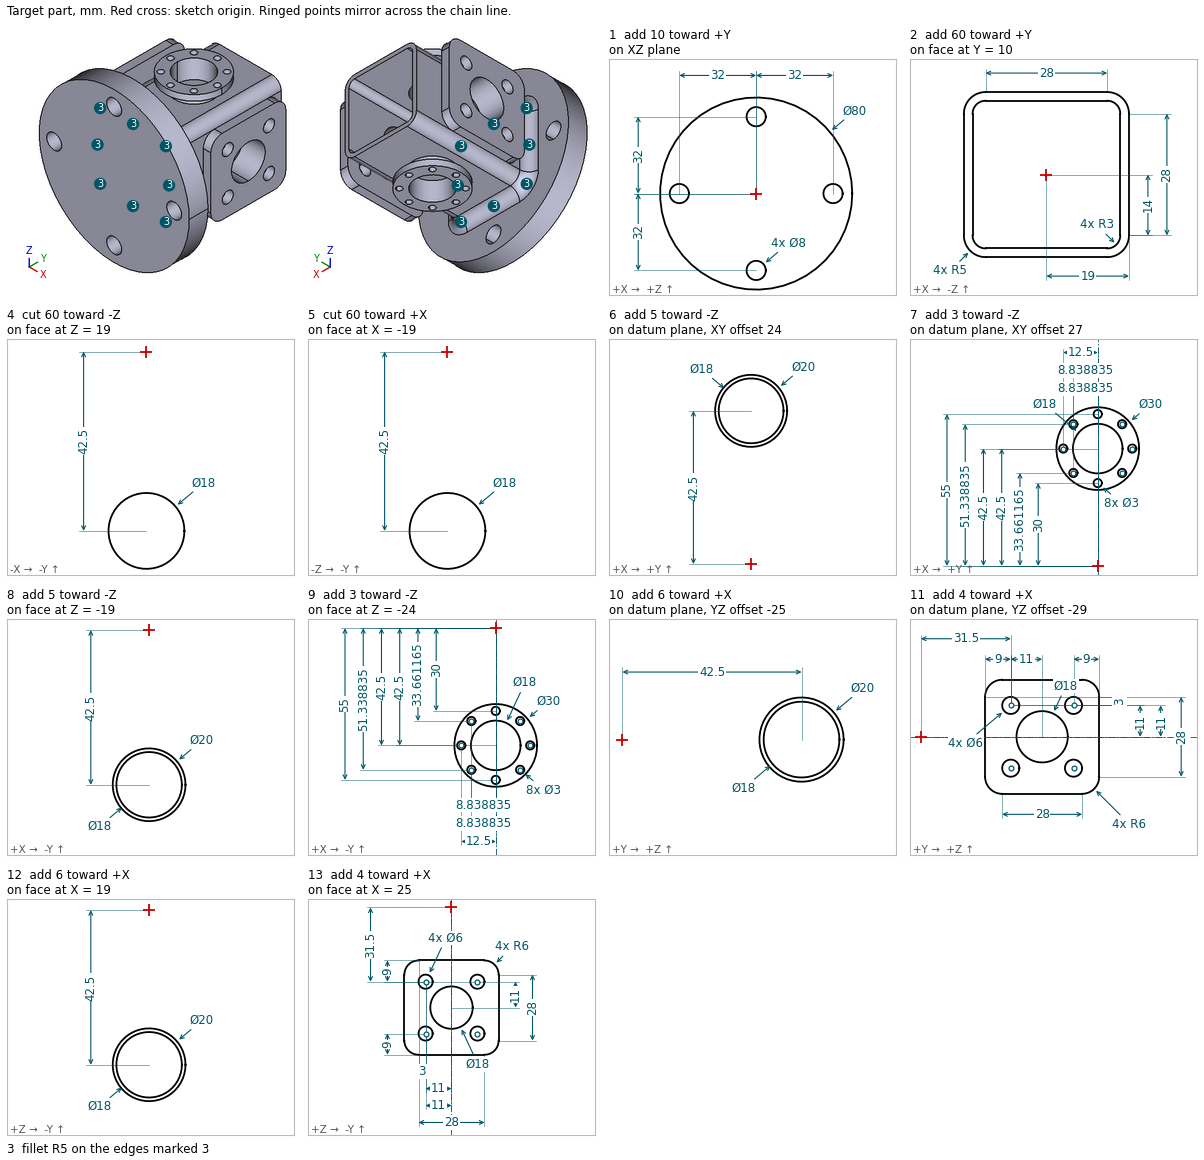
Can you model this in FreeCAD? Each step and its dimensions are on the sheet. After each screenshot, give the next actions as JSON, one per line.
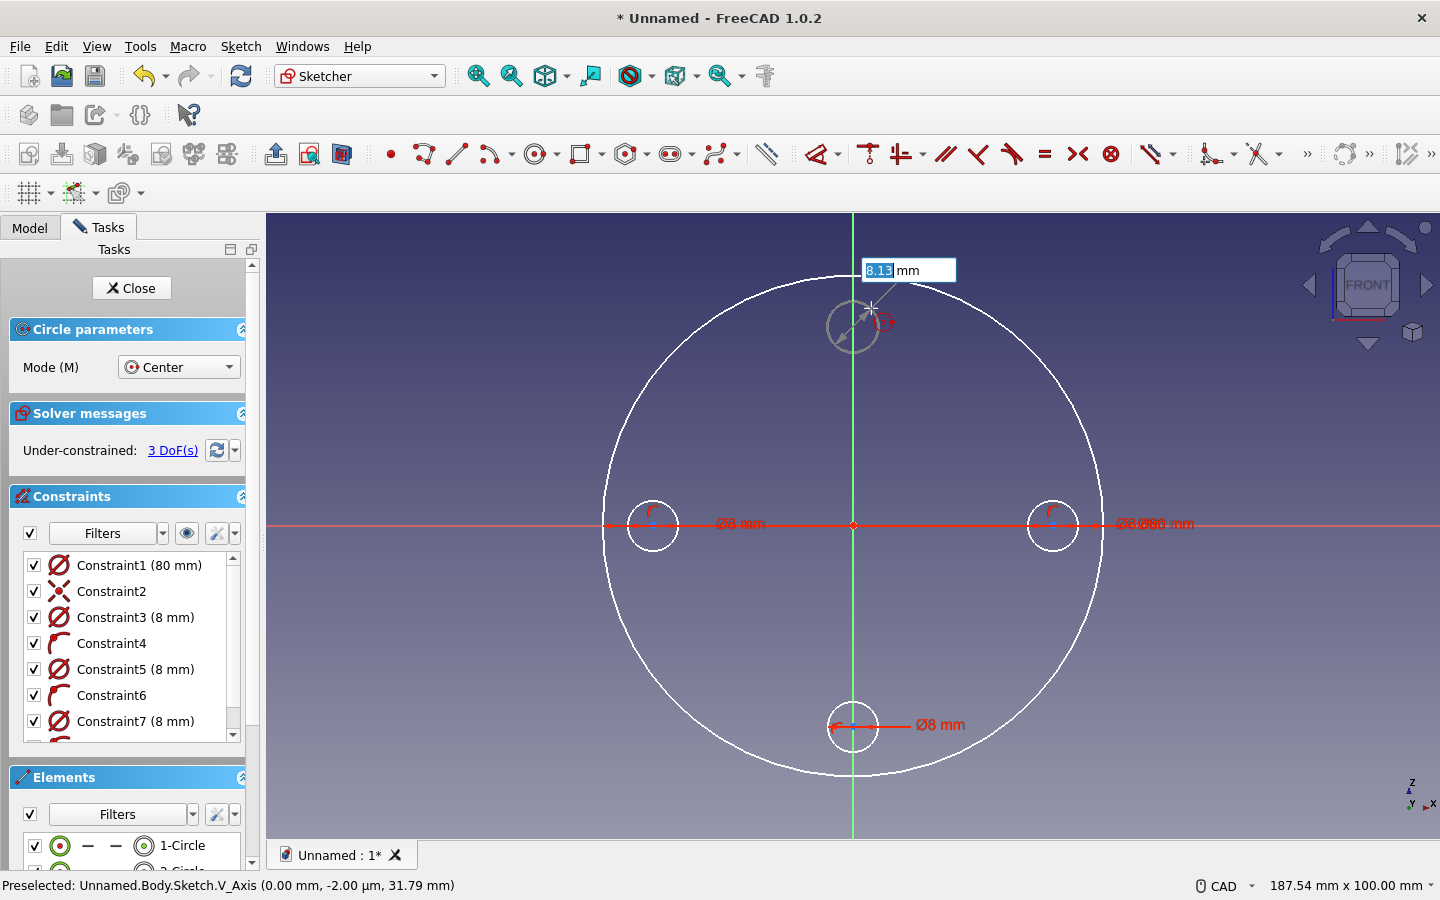
{"action": "type", "text": "8"}
{"action": "key", "text": "Return"}
{"action": "key", "text": "Escape"}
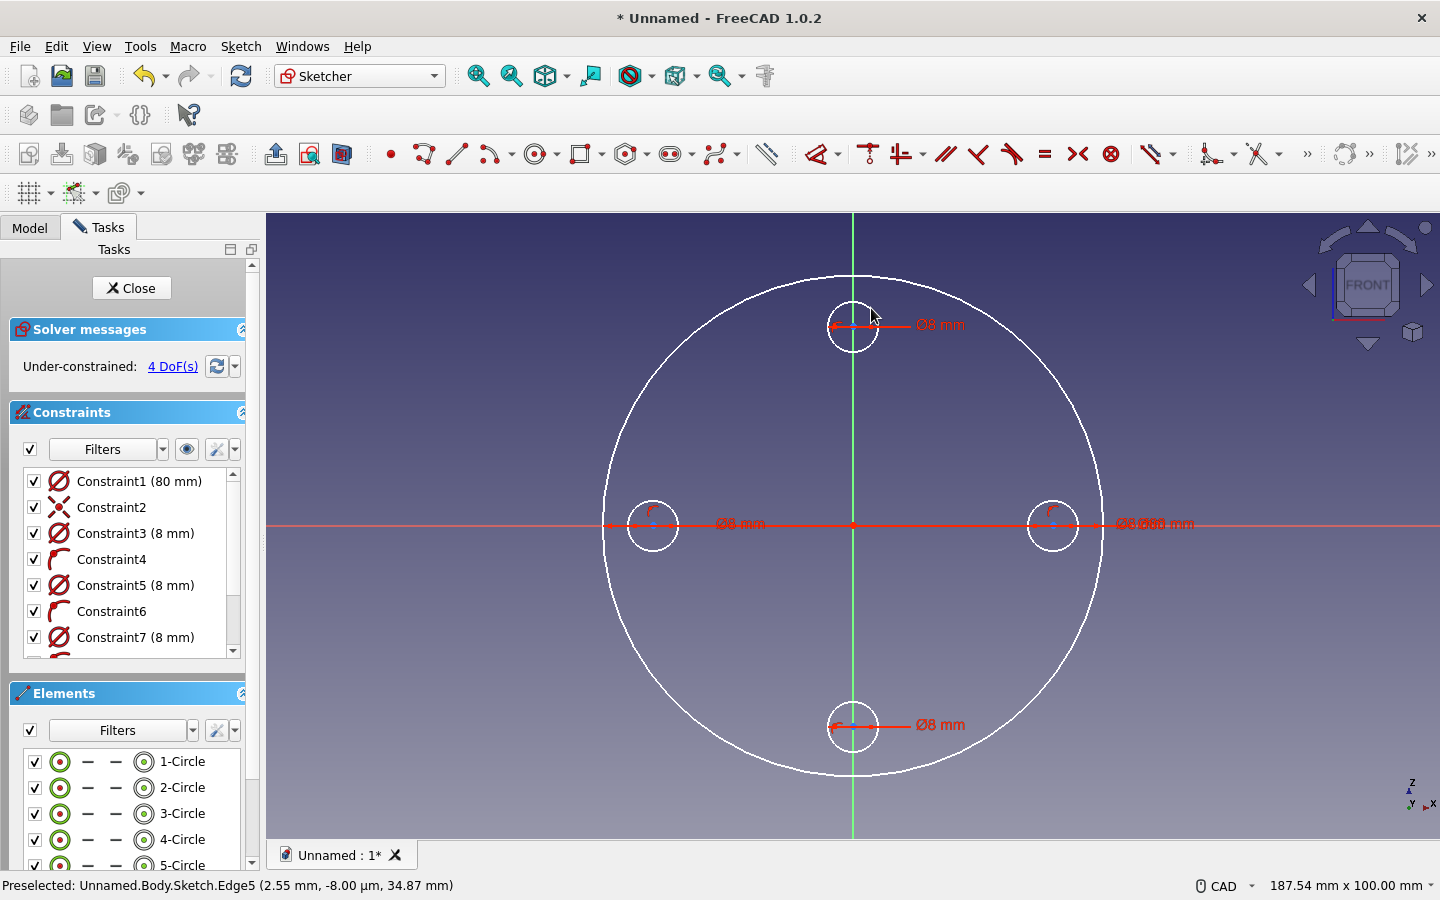
{"action": "left_click", "coordinate": [853, 727]}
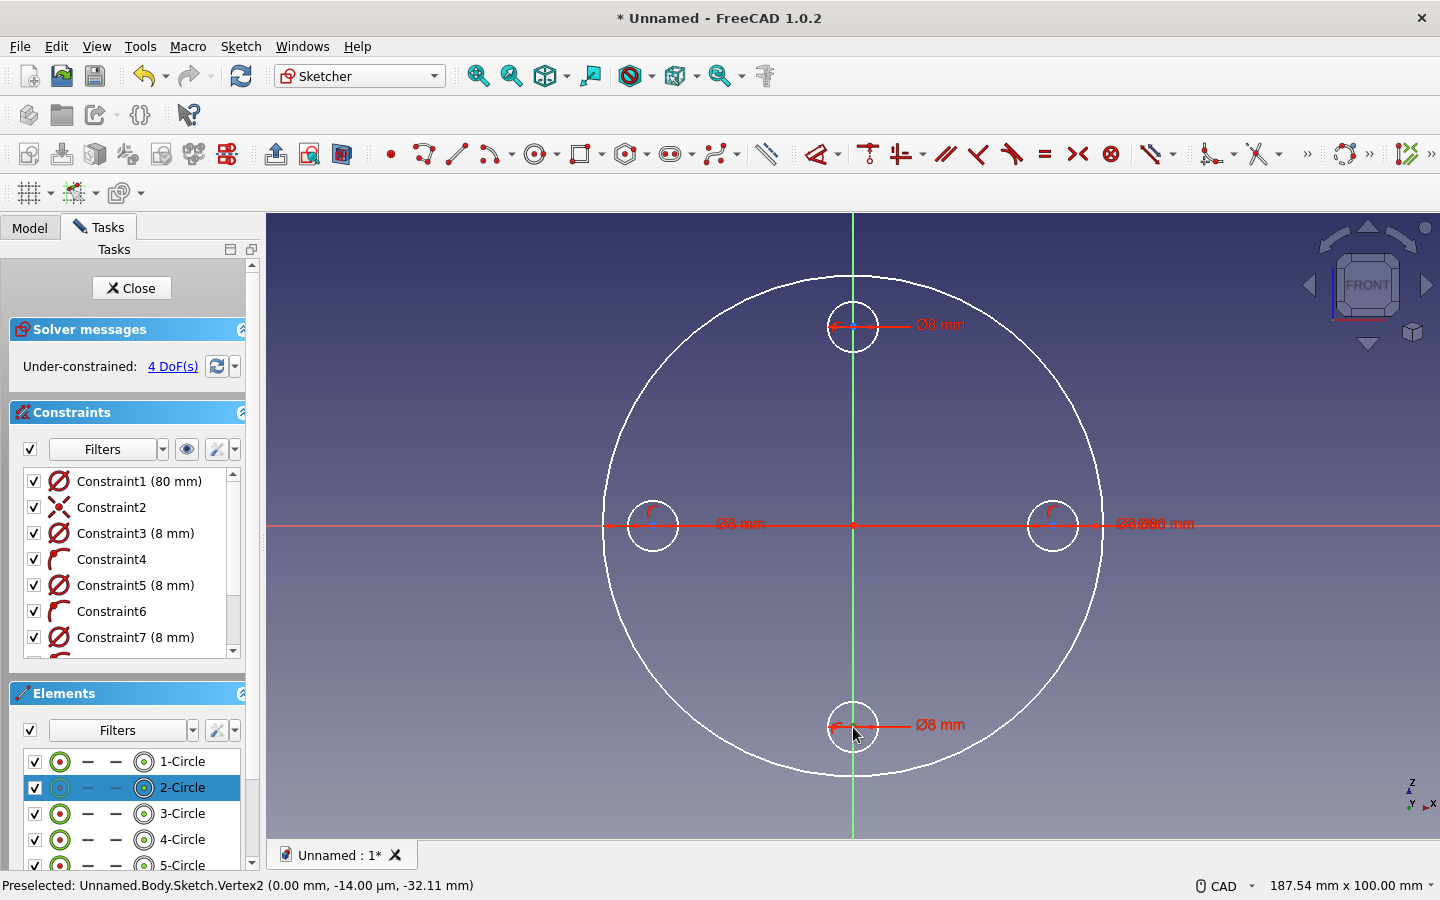
{"action": "left_click", "coordinate": [838, 154]}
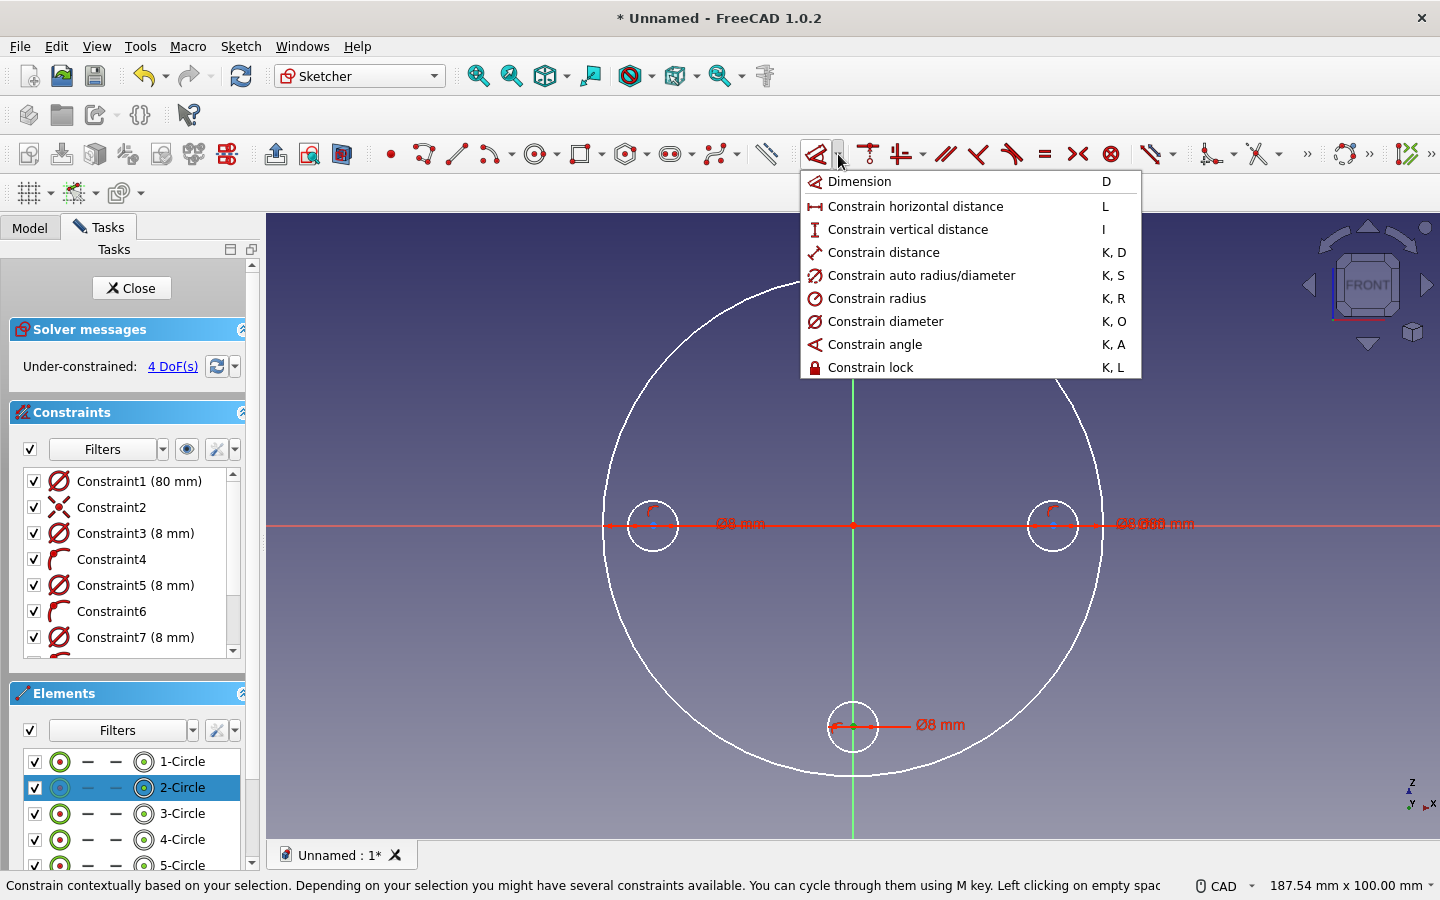
{"action": "left_click", "coordinate": [971, 230]}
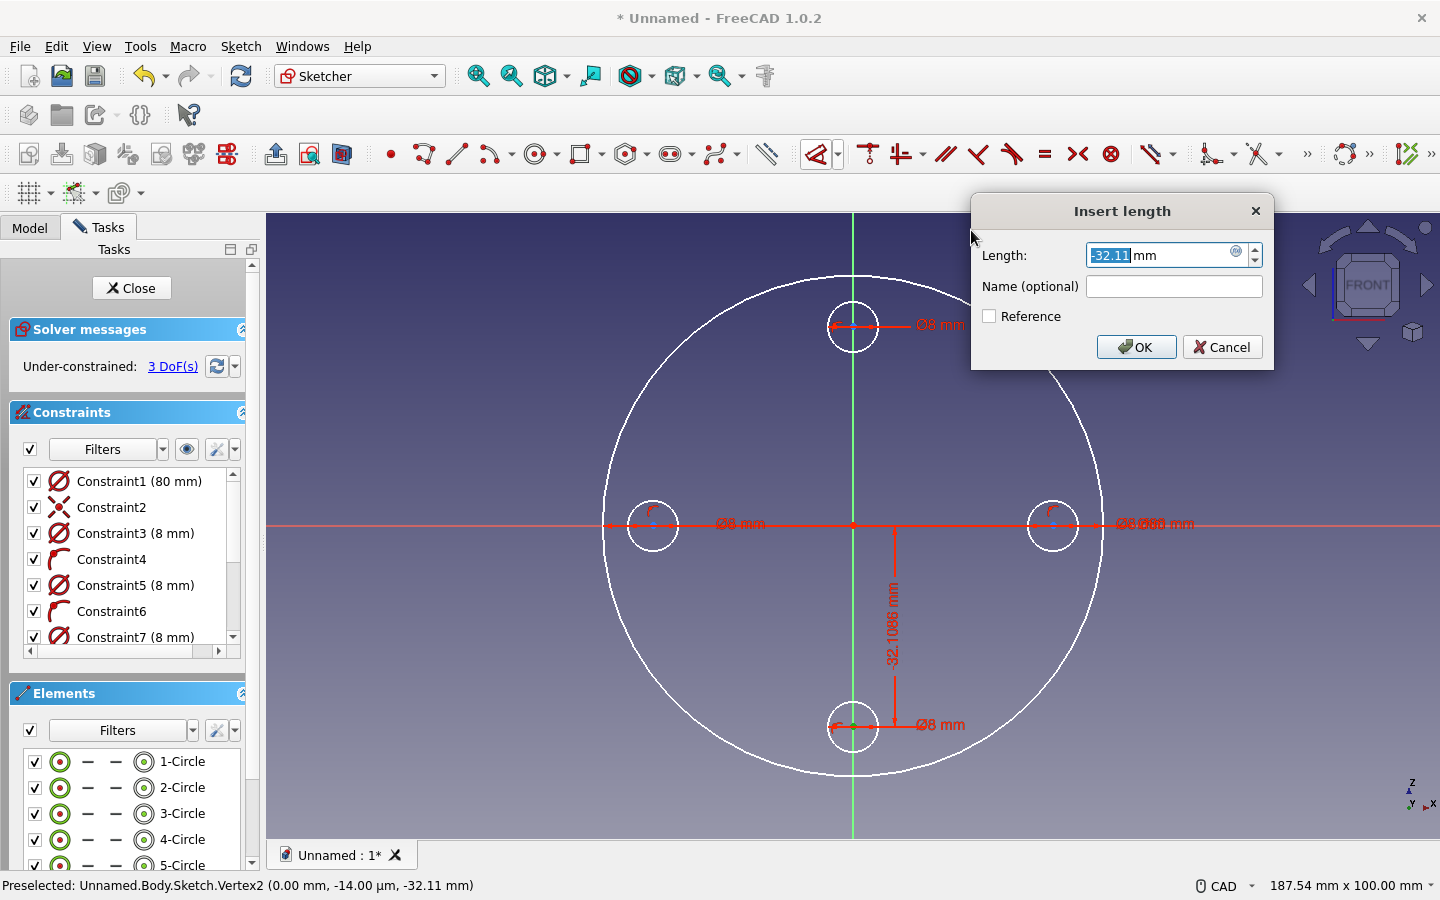
{"action": "type", "text": "-32"}
{"action": "key", "text": "Return"}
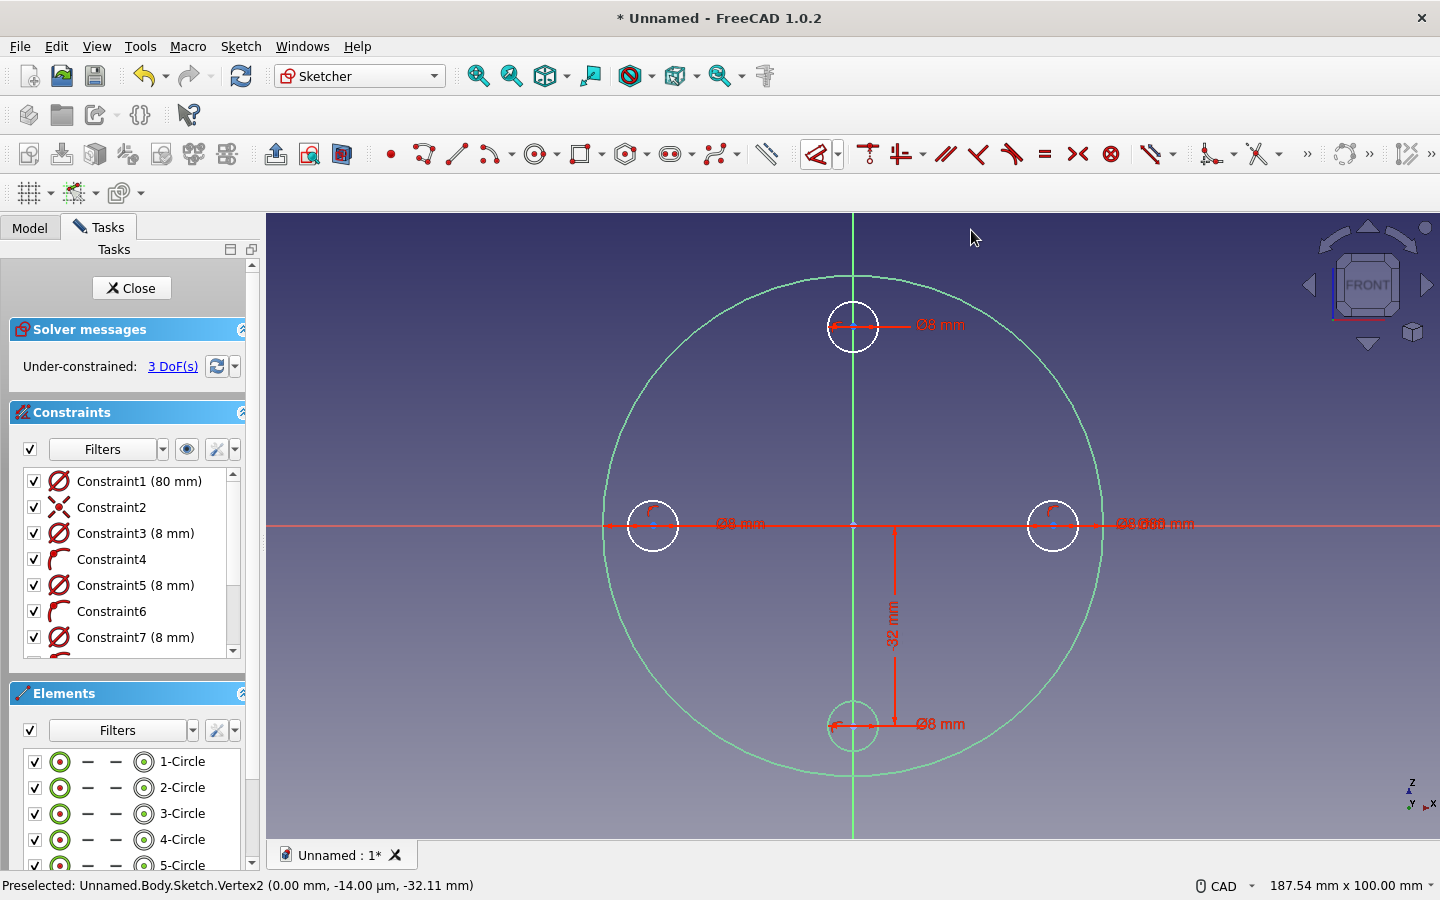
{"action": "left_click", "coordinate": [653, 526]}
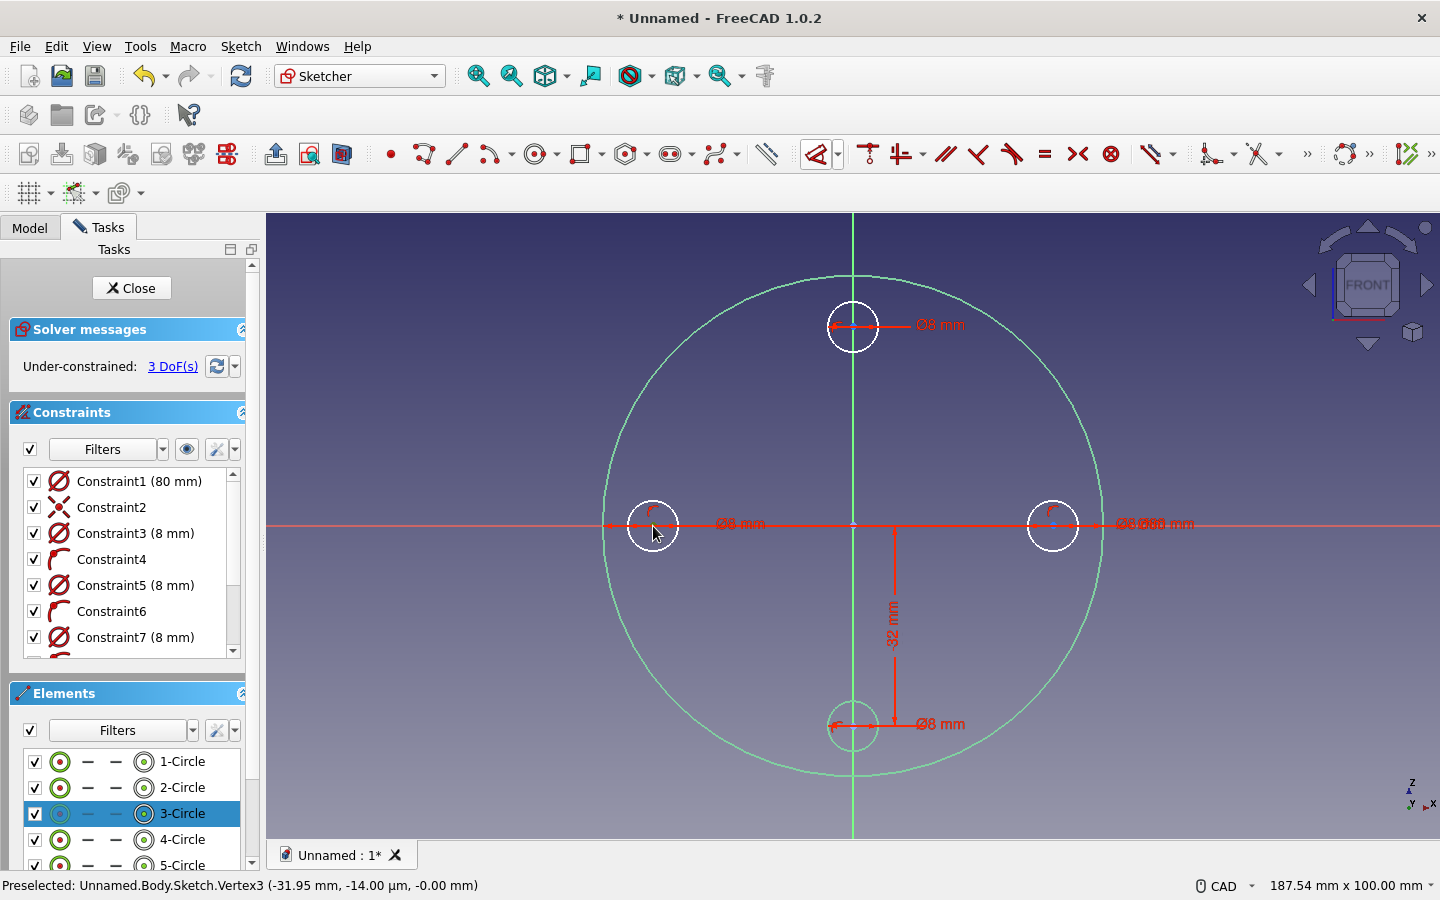
{"action": "key", "text": "l"}